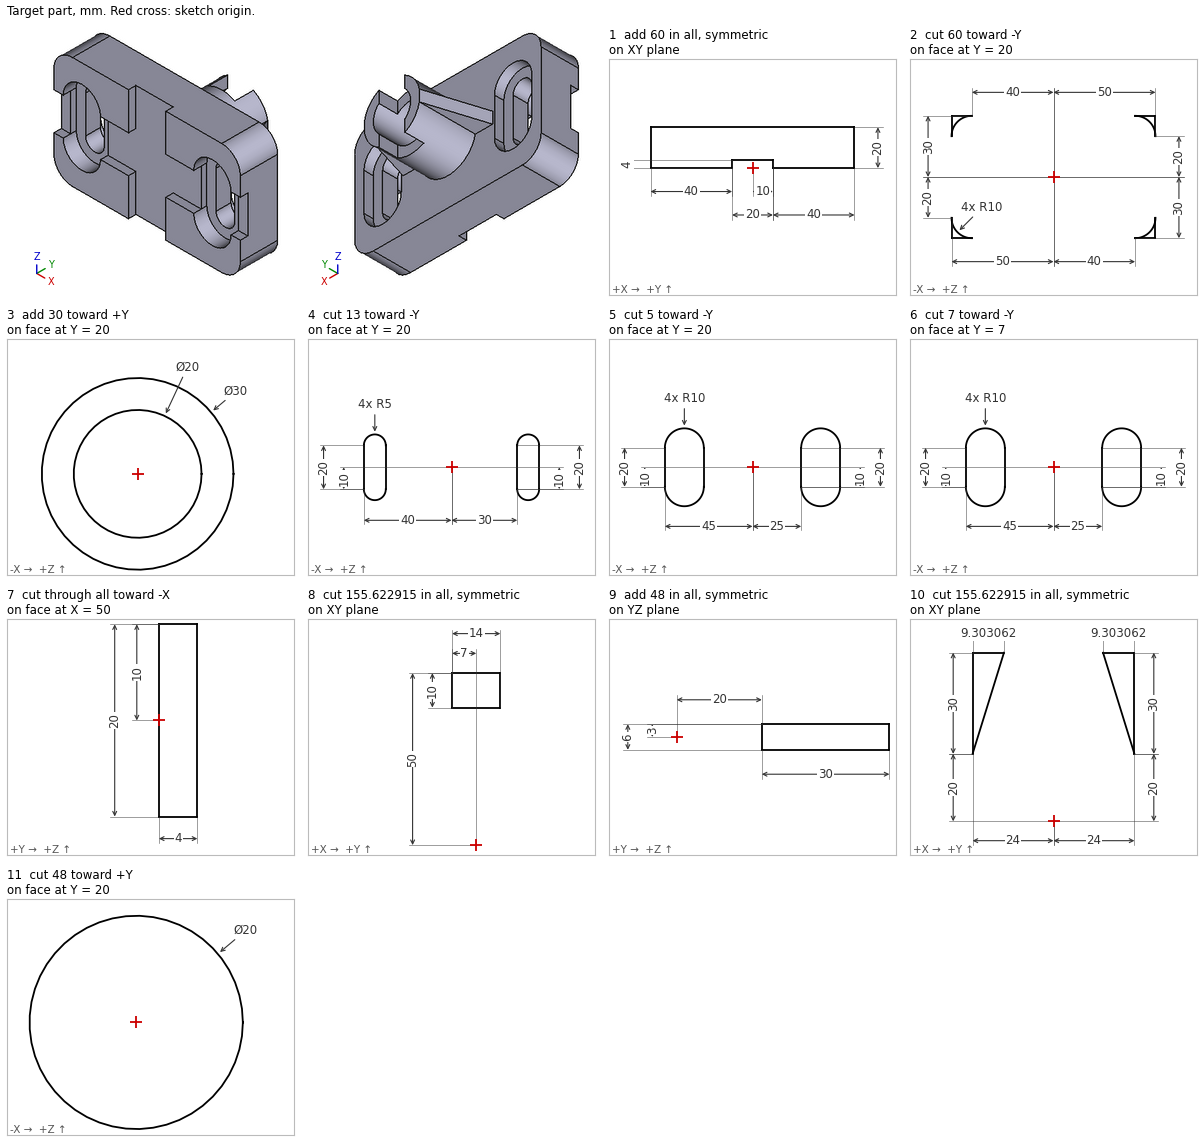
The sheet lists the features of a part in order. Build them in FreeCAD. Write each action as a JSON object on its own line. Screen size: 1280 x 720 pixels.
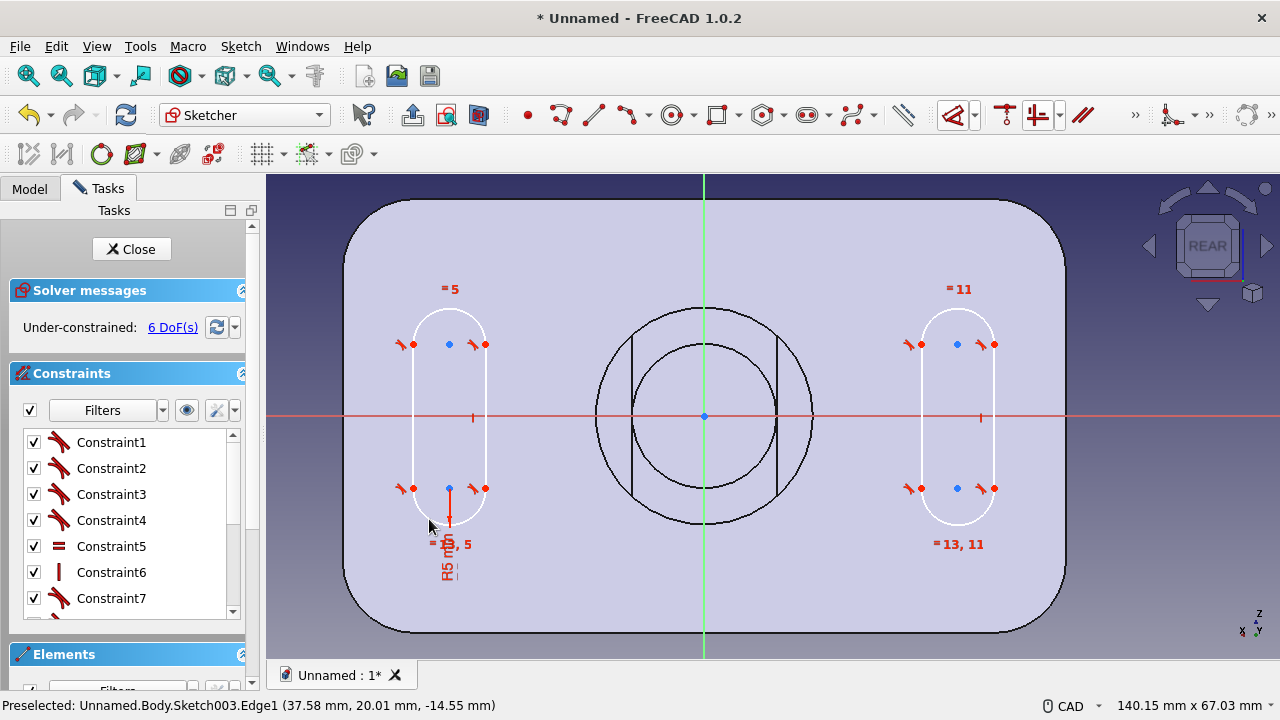
{"action": "left_click", "coordinate": [413, 446]}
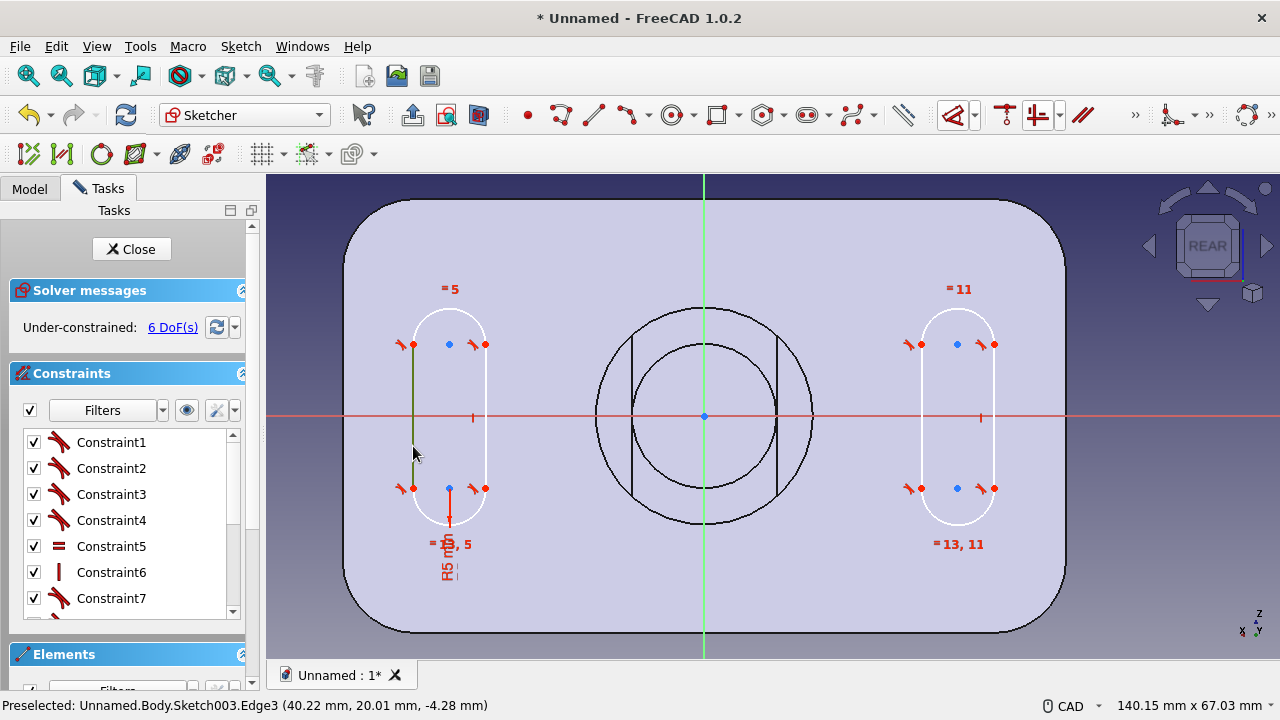
{"action": "key", "text": "i"}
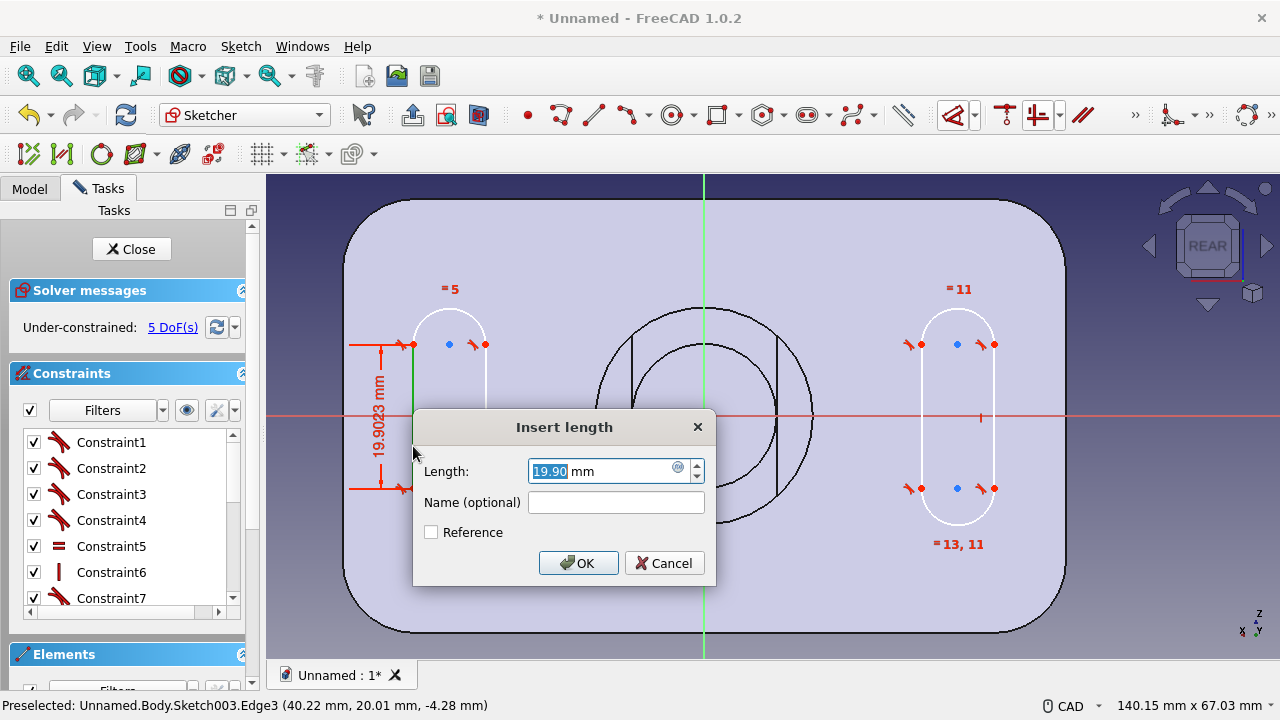
{"action": "type", "text": "20"}
{"action": "key", "text": "Return"}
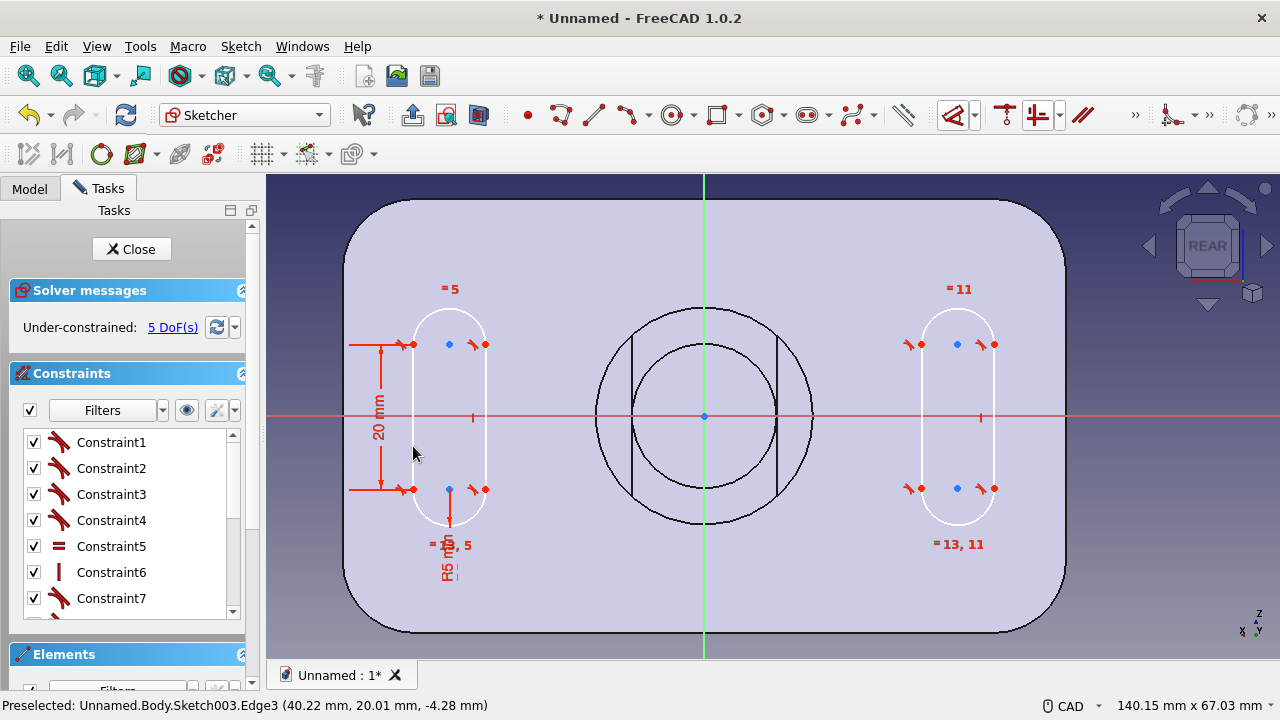
{"action": "left_click", "coordinate": [922, 446]}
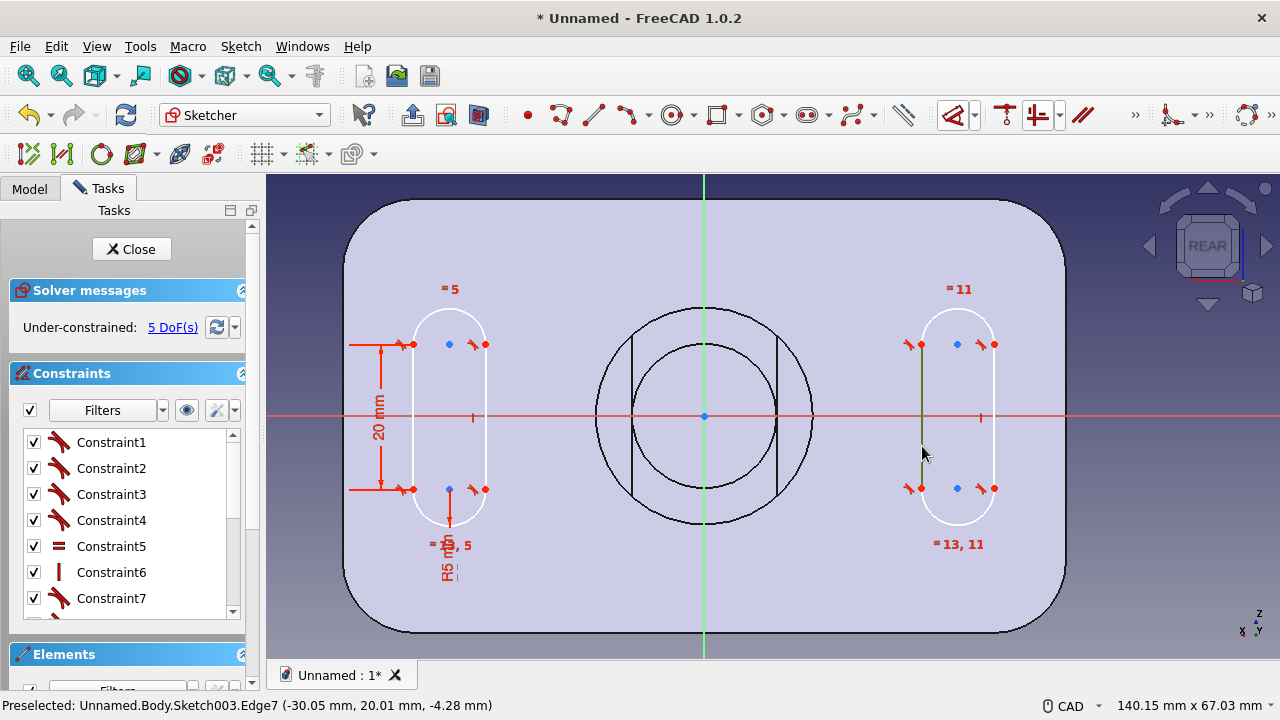
{"action": "key", "text": "i"}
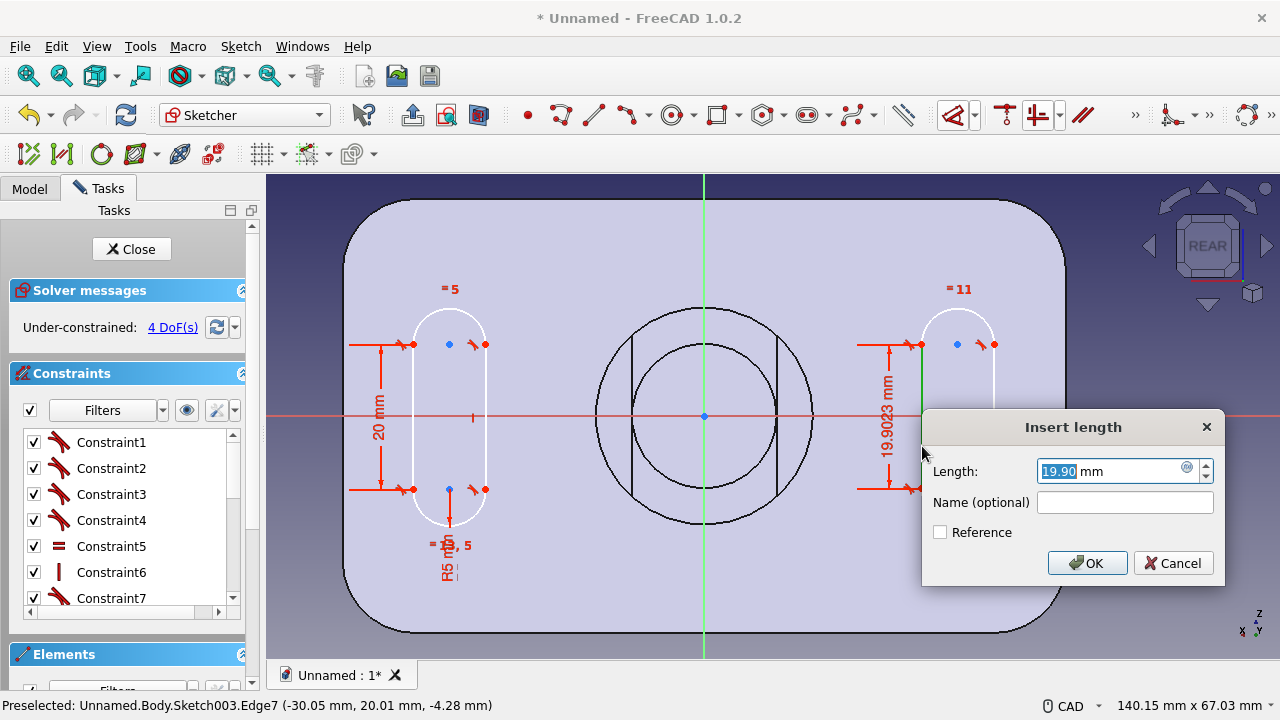
{"action": "type", "text": "20"}
{"action": "key", "text": "Return"}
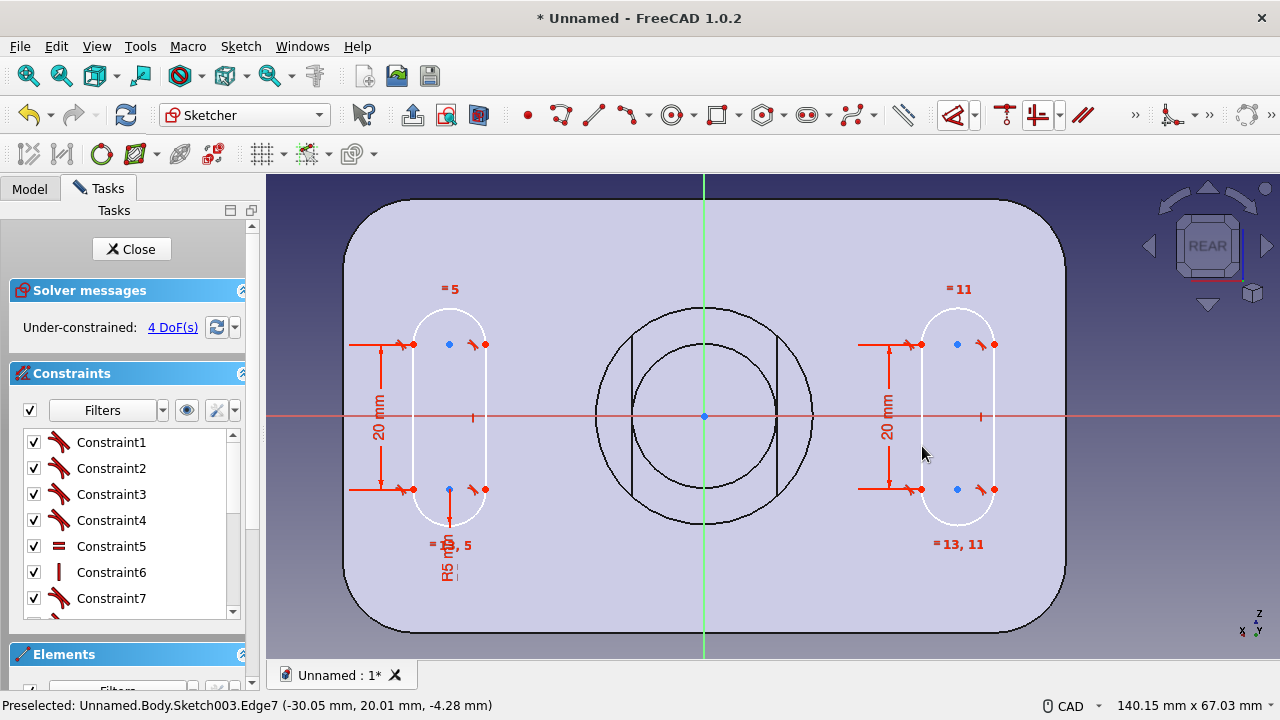
{"action": "left_click", "coordinate": [413, 490]}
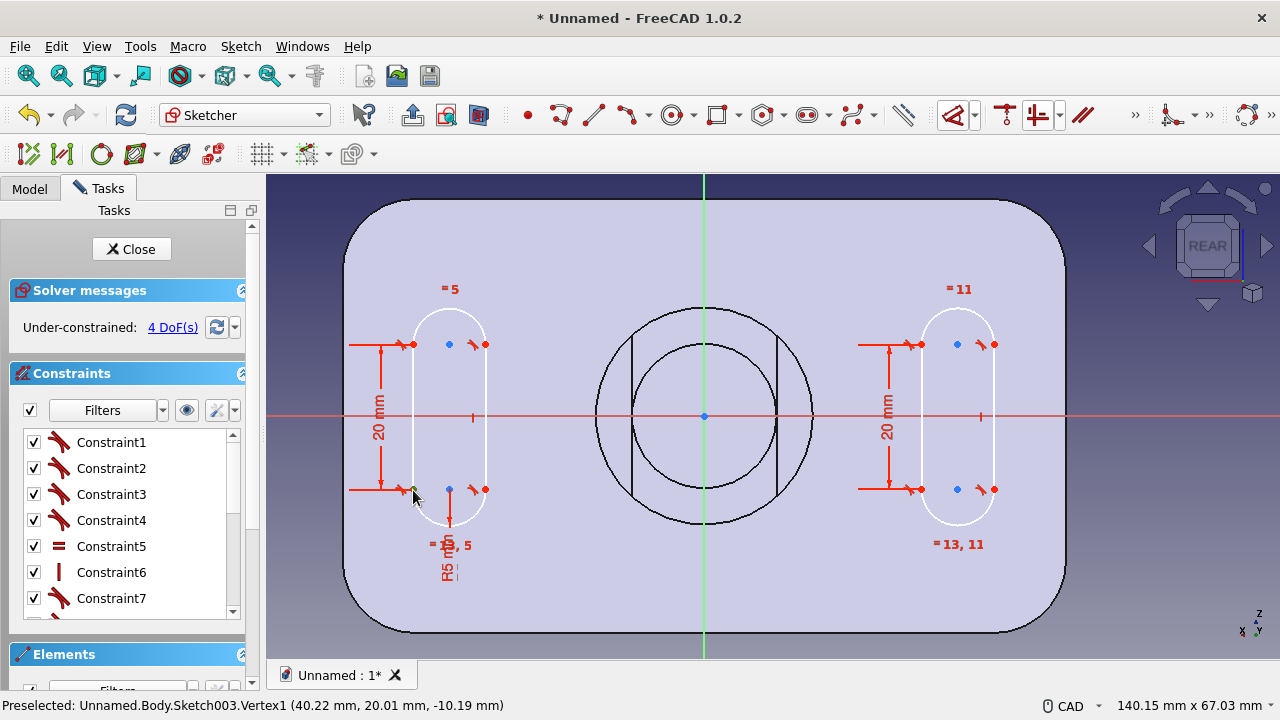
{"action": "key", "text": "l"}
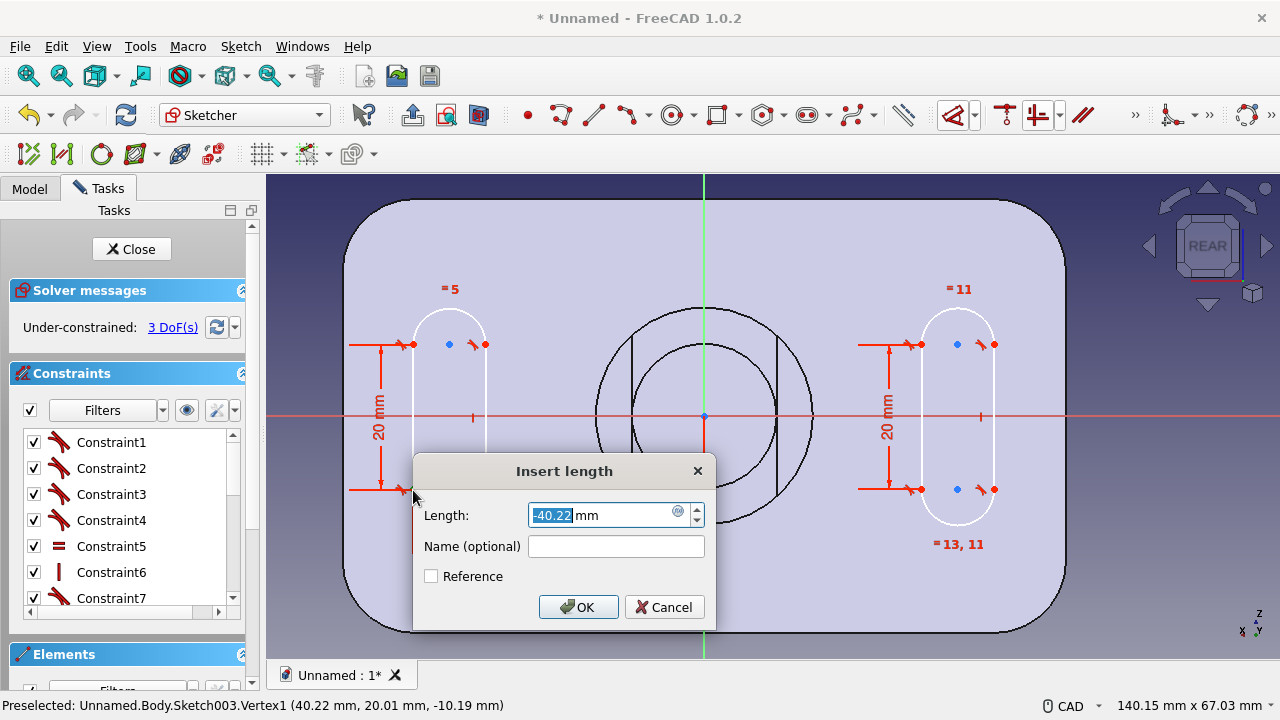
{"action": "type", "text": "-40"}
{"action": "key", "text": "Return"}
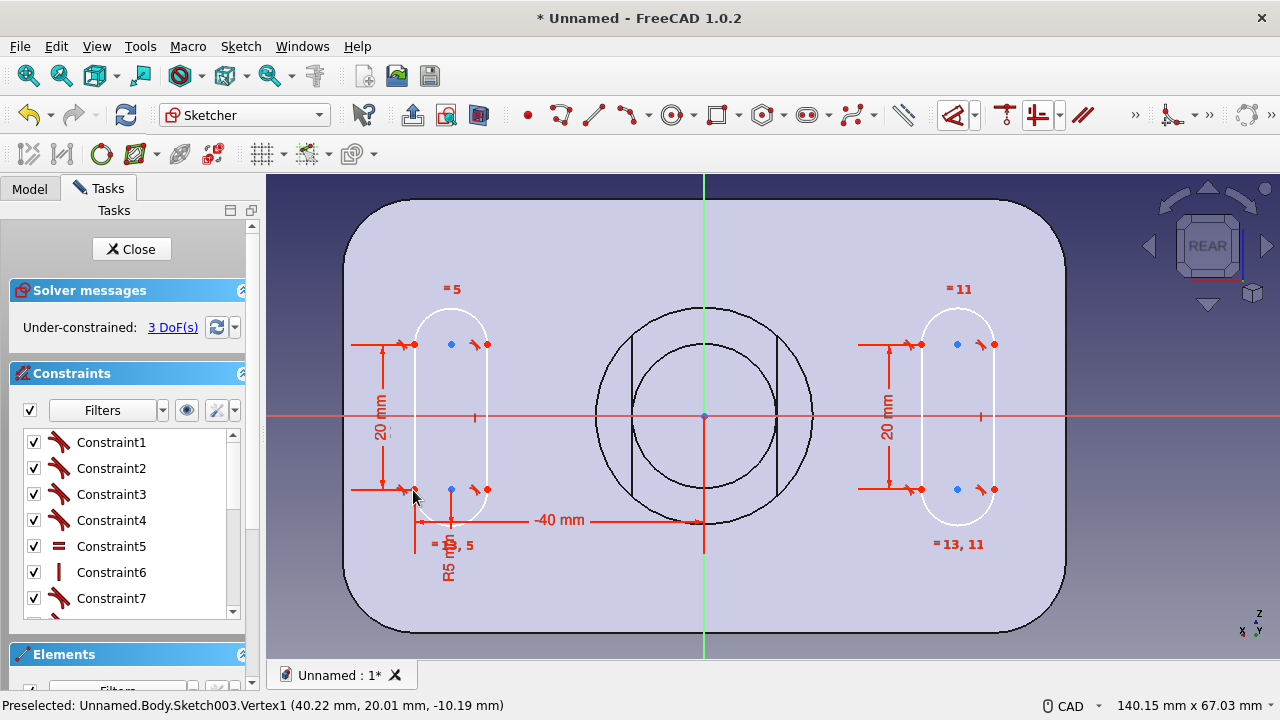
{"action": "left_click", "coordinate": [415, 490]}